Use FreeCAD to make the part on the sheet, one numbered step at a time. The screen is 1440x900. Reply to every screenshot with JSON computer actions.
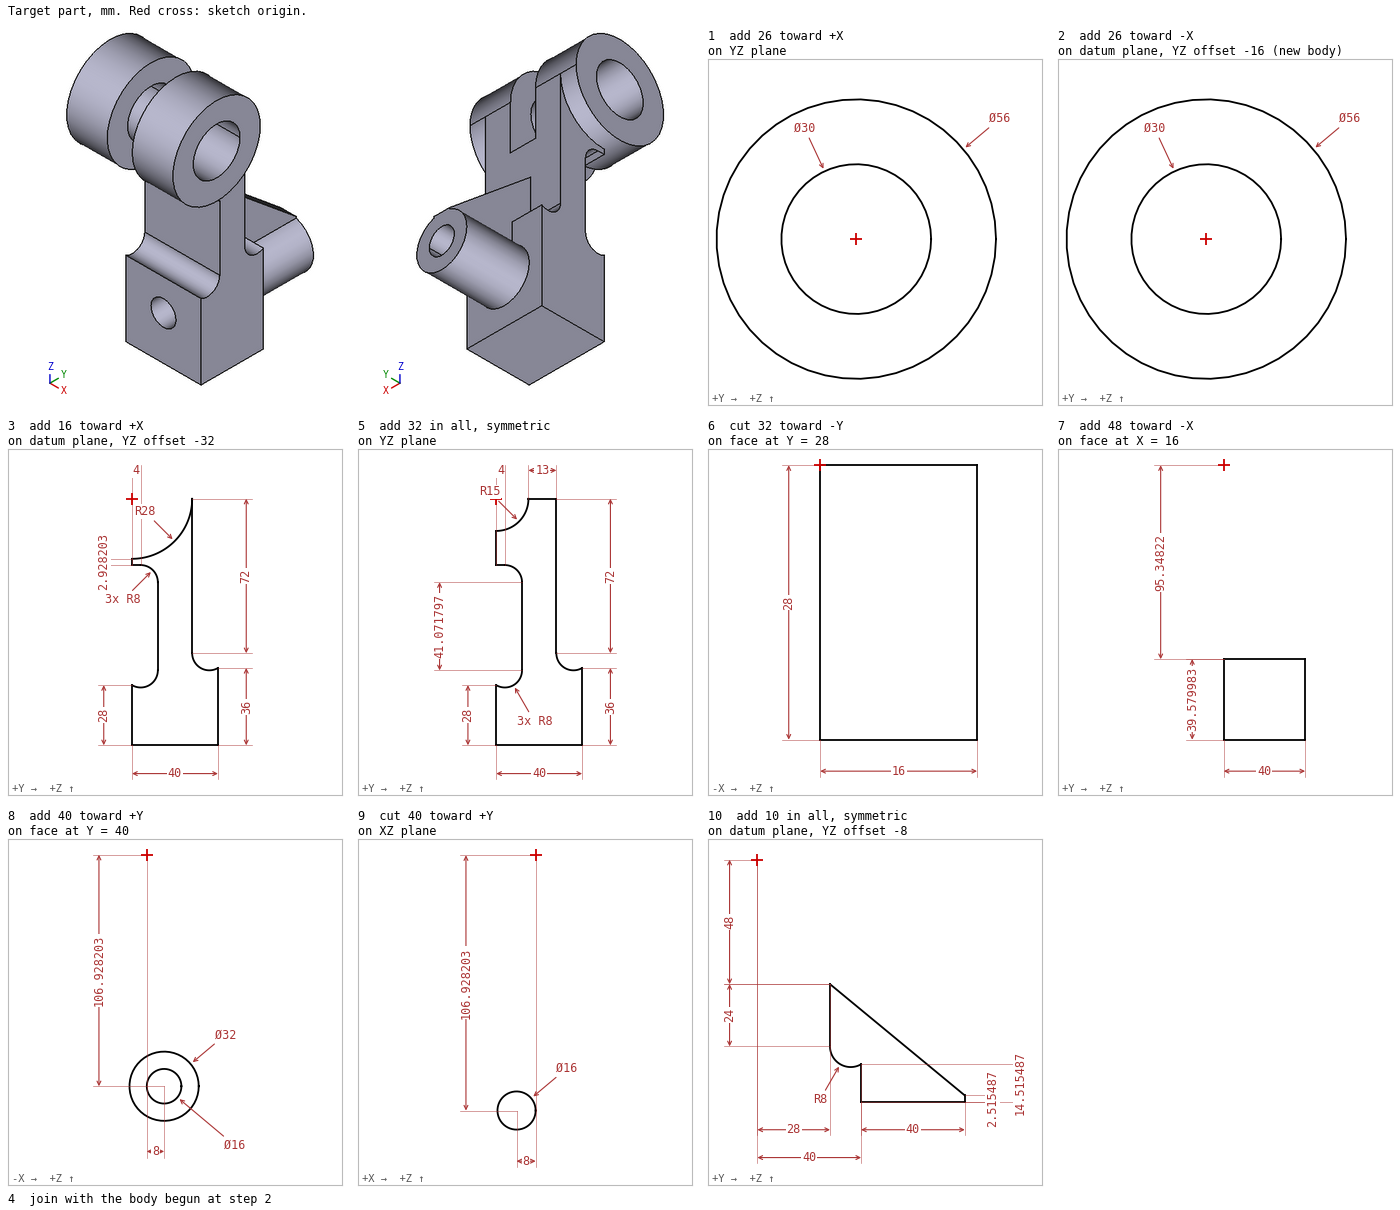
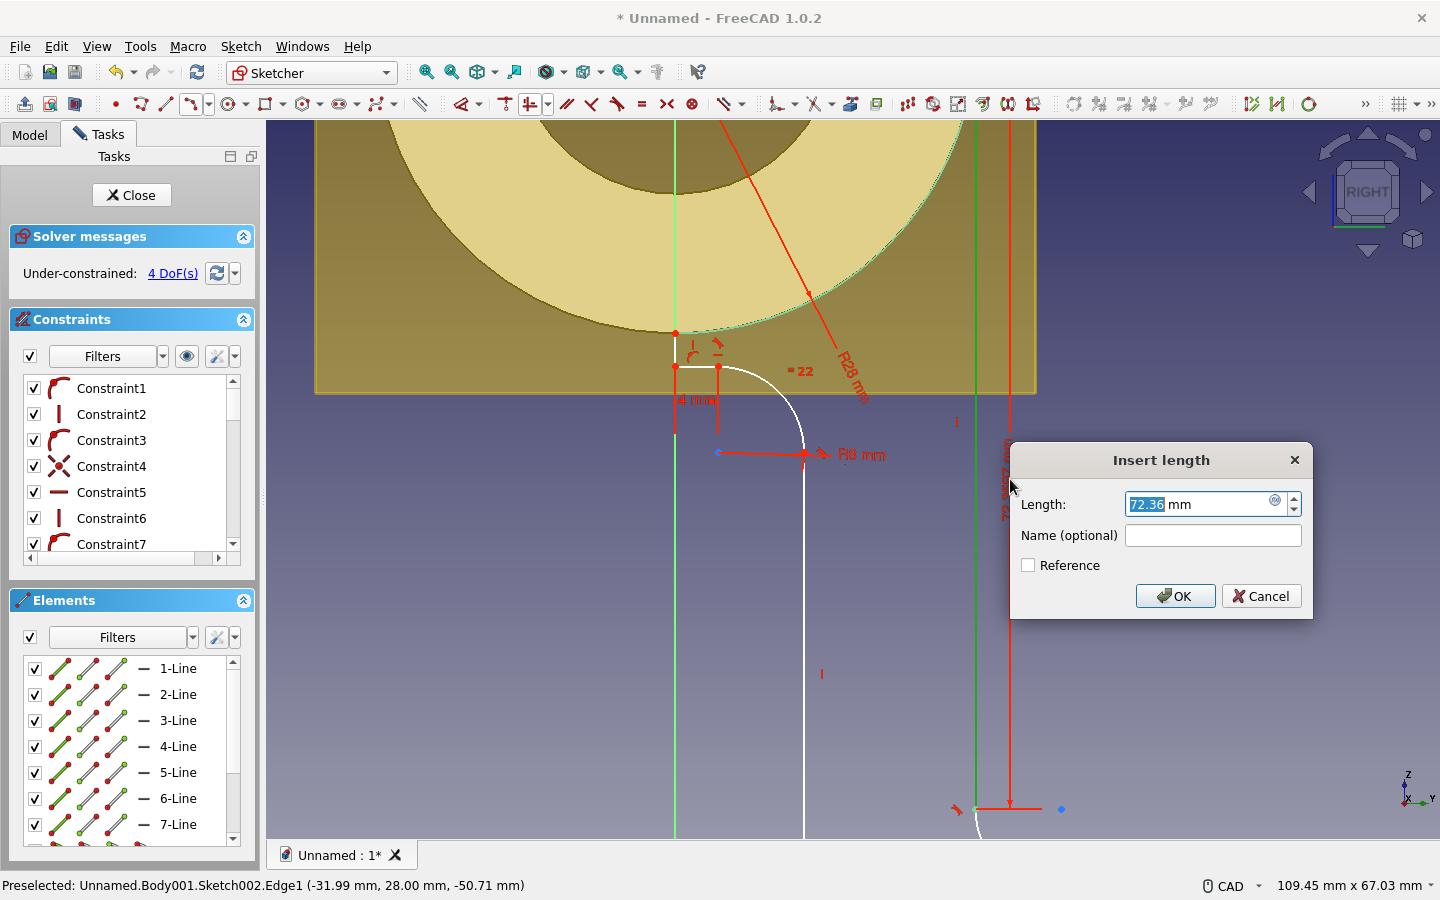
{"action": "type", "text": "72"}
{"action": "key", "text": "Return"}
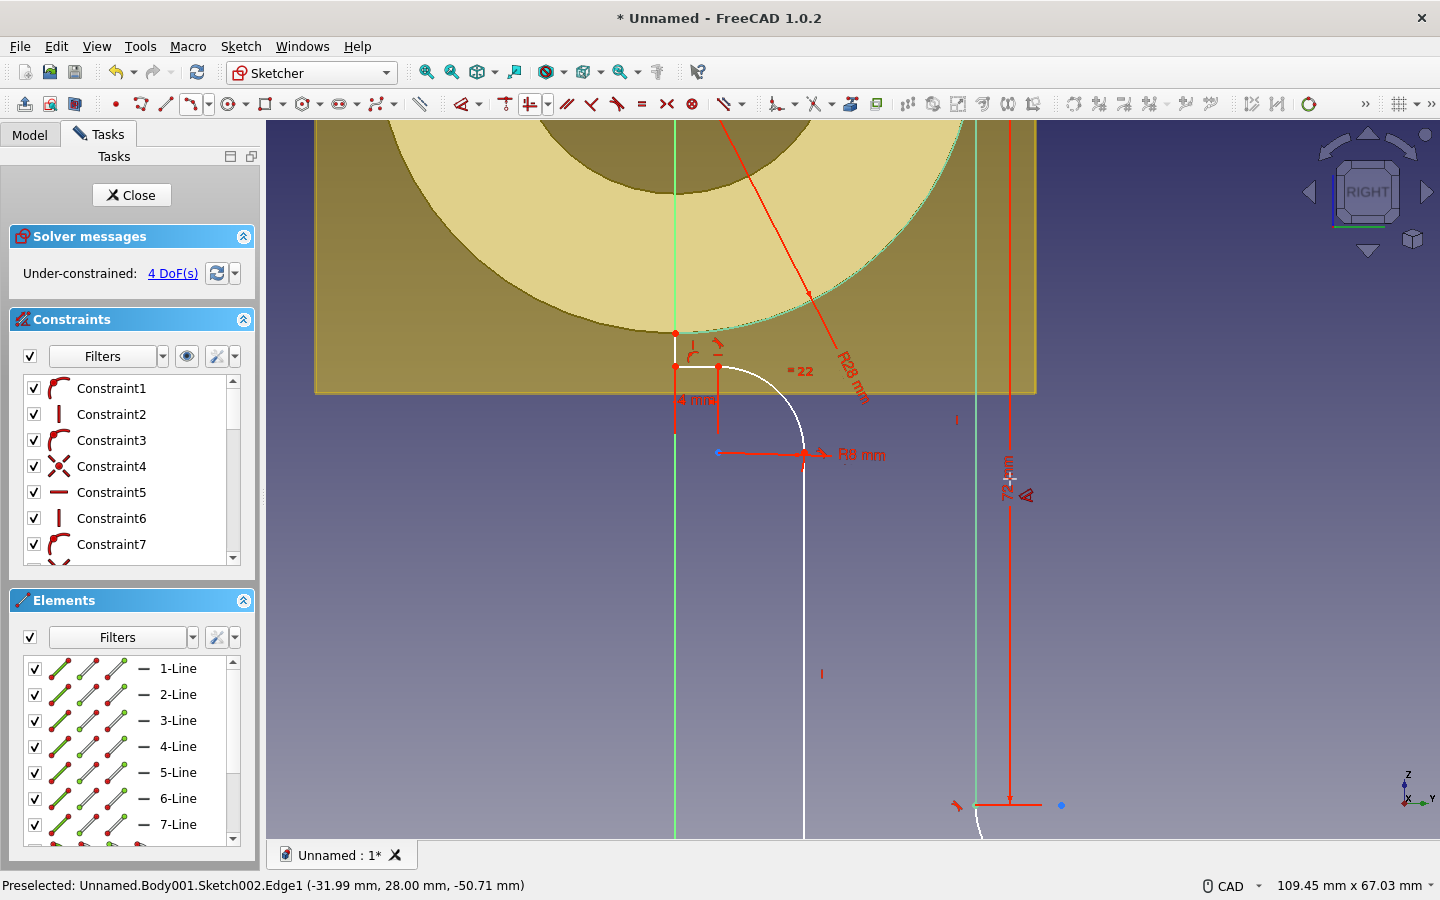
{"action": "scroll", "coordinate": [723, 381], "scroll_direction": "down", "scroll_amount": 5}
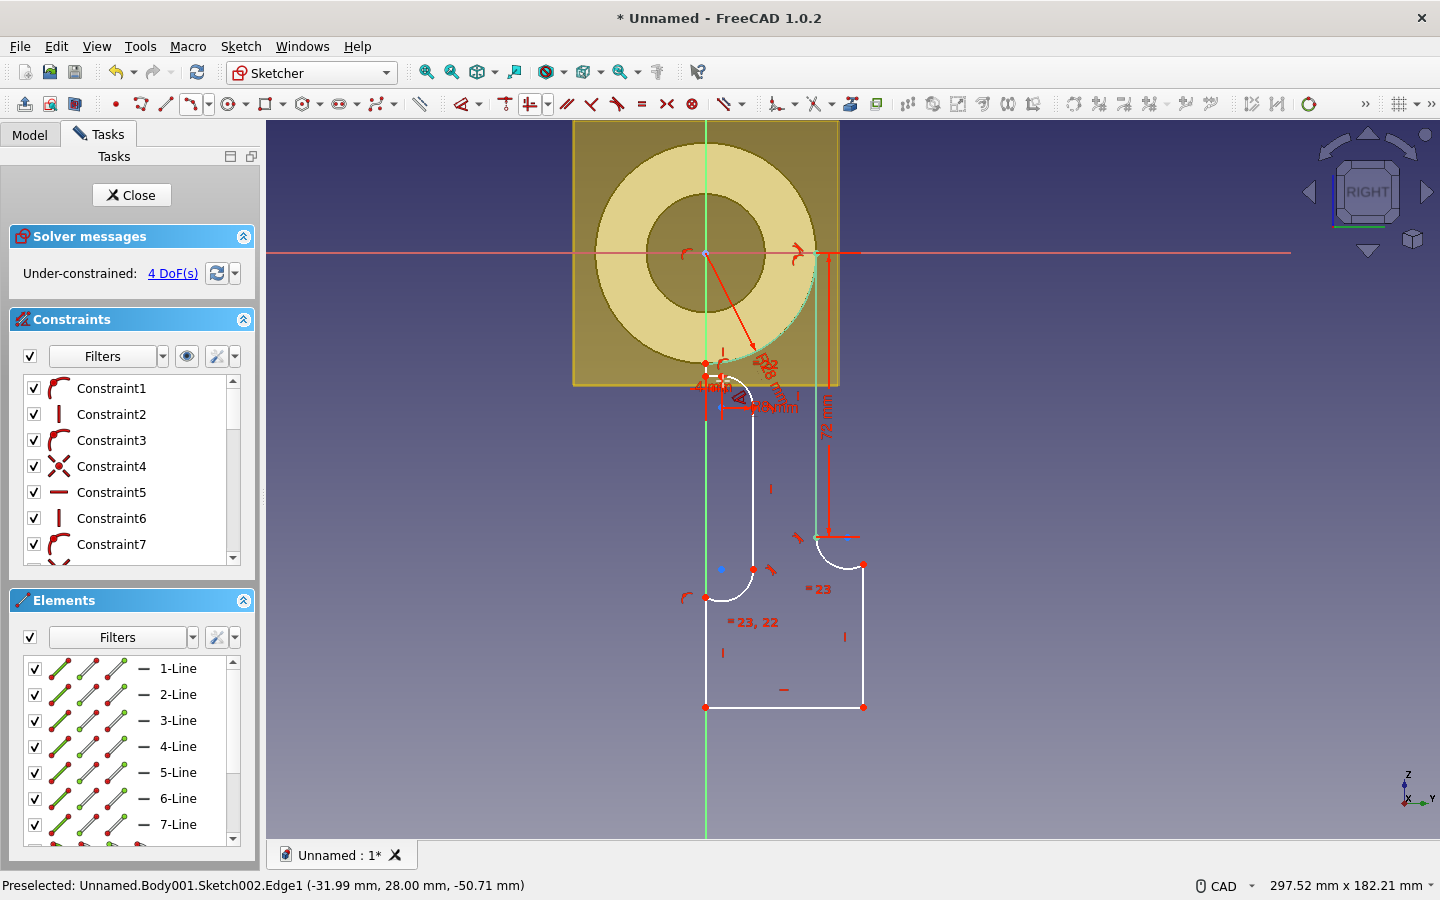
{"action": "left_click", "coordinate": [706, 630]}
{"action": "left_click", "coordinate": [672, 652]}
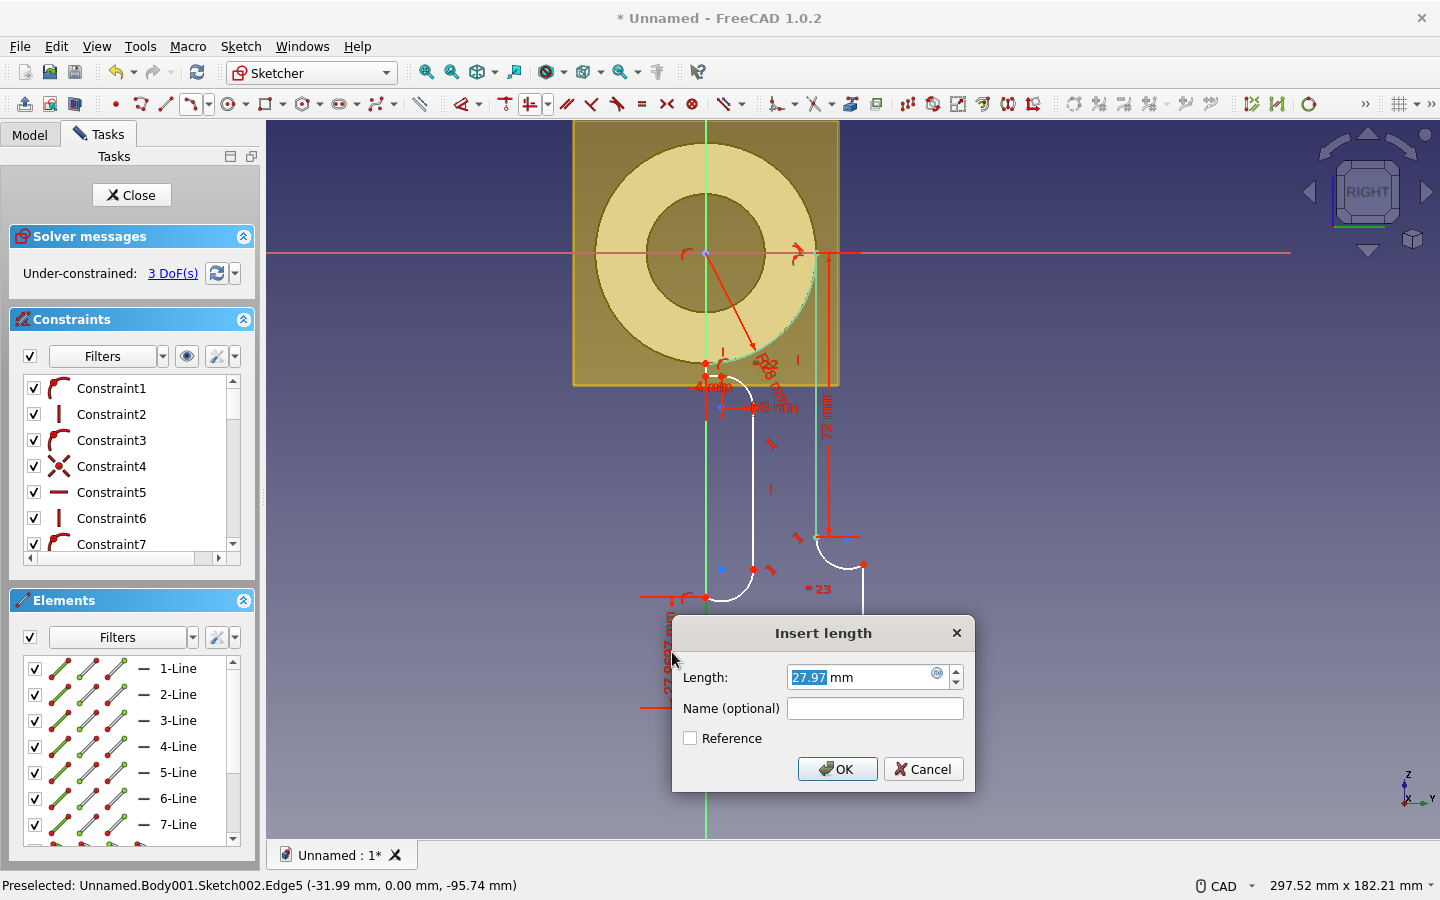
{"action": "type", "text": "28"}
{"action": "key", "text": "Return"}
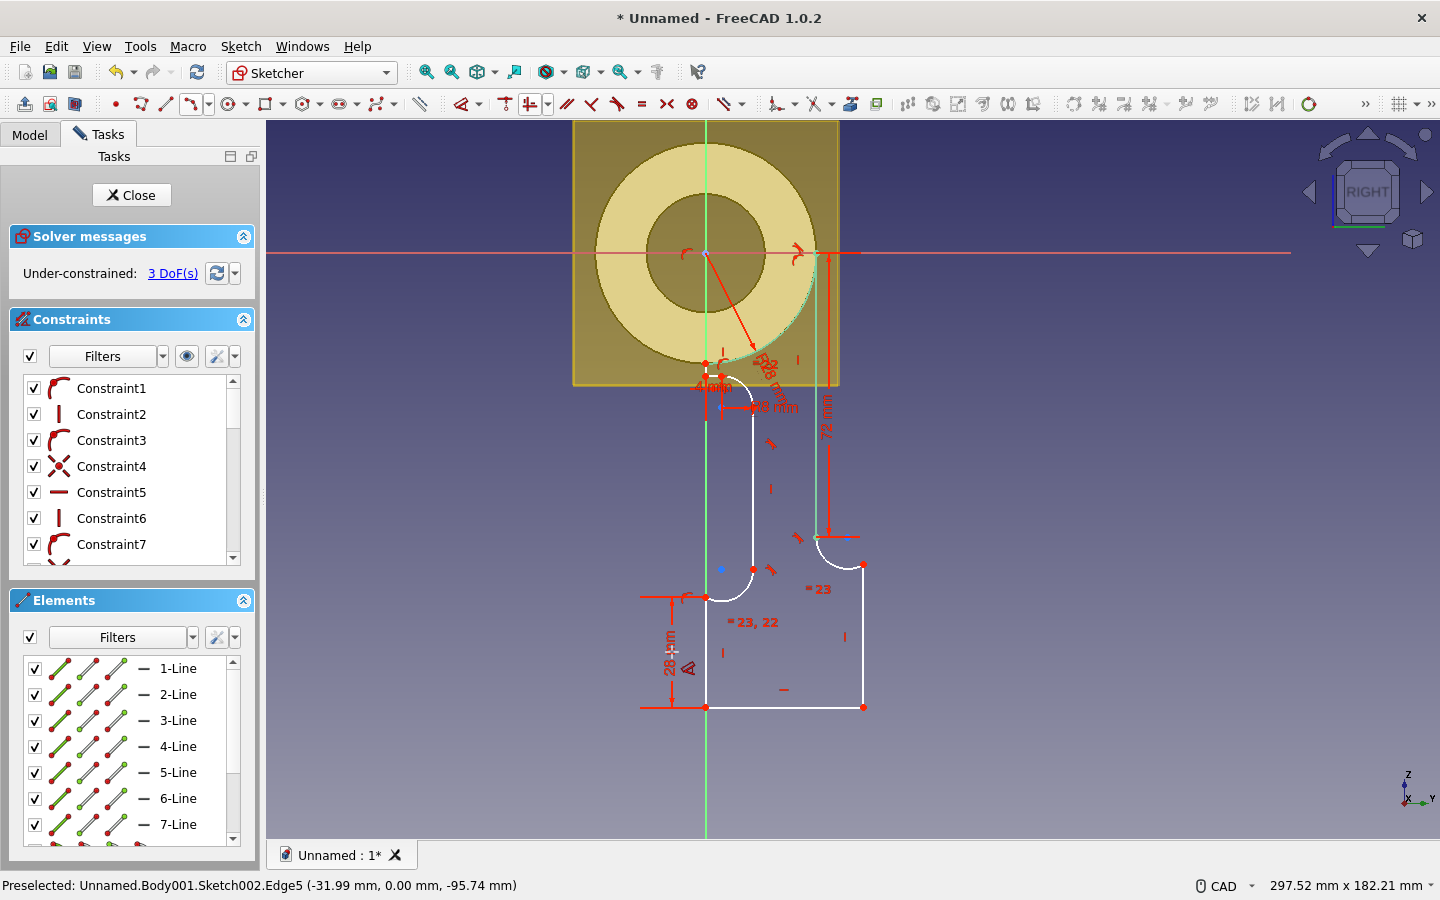
{"action": "left_click", "coordinate": [753, 708]}
{"action": "left_click", "coordinate": [784, 742]}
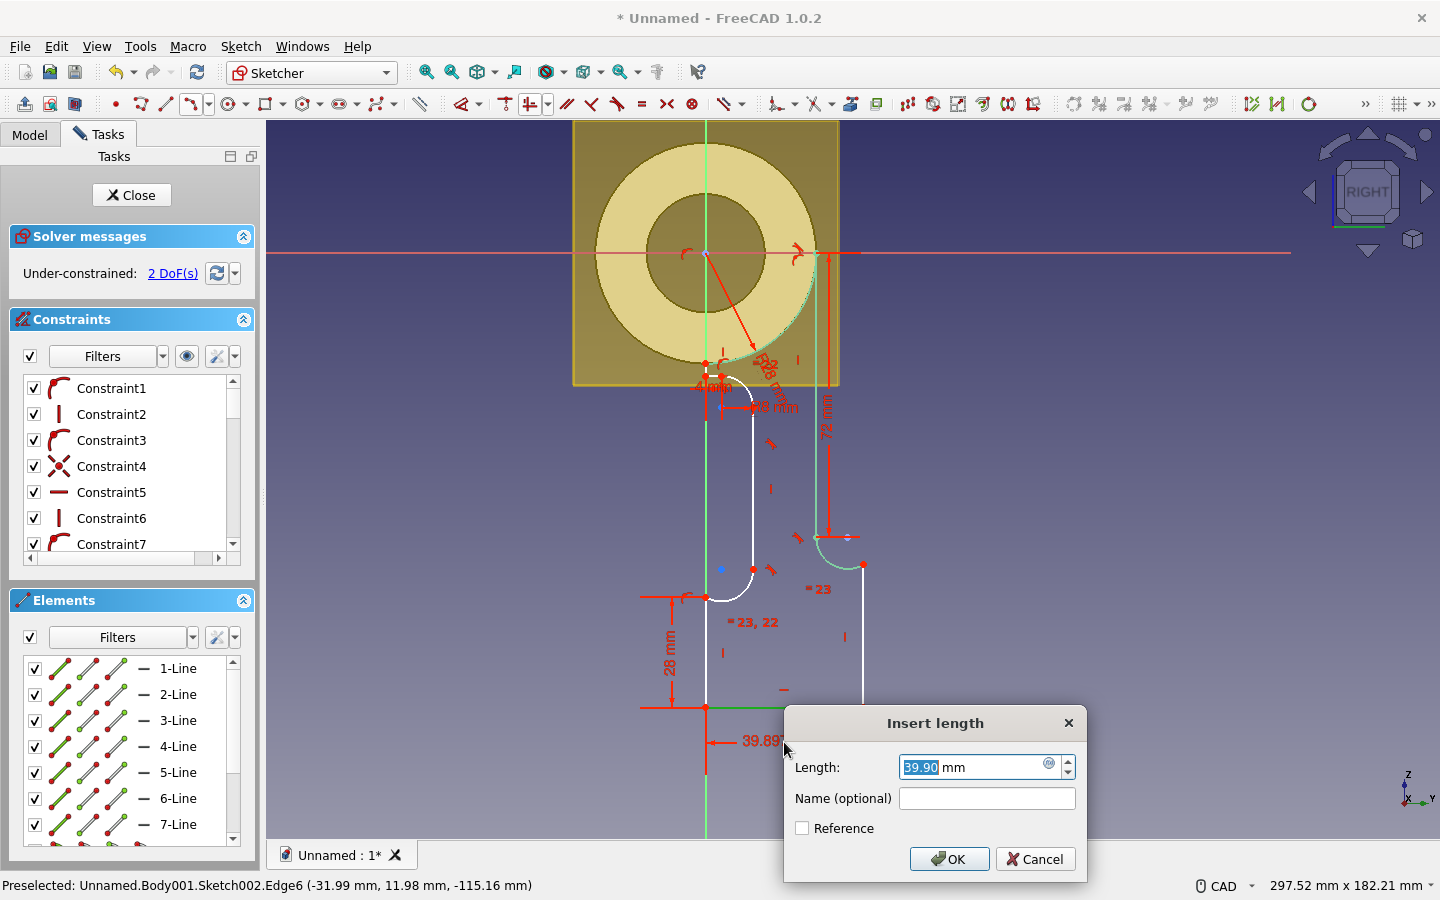
{"action": "type", "text": "40"}
{"action": "key", "text": "Return"}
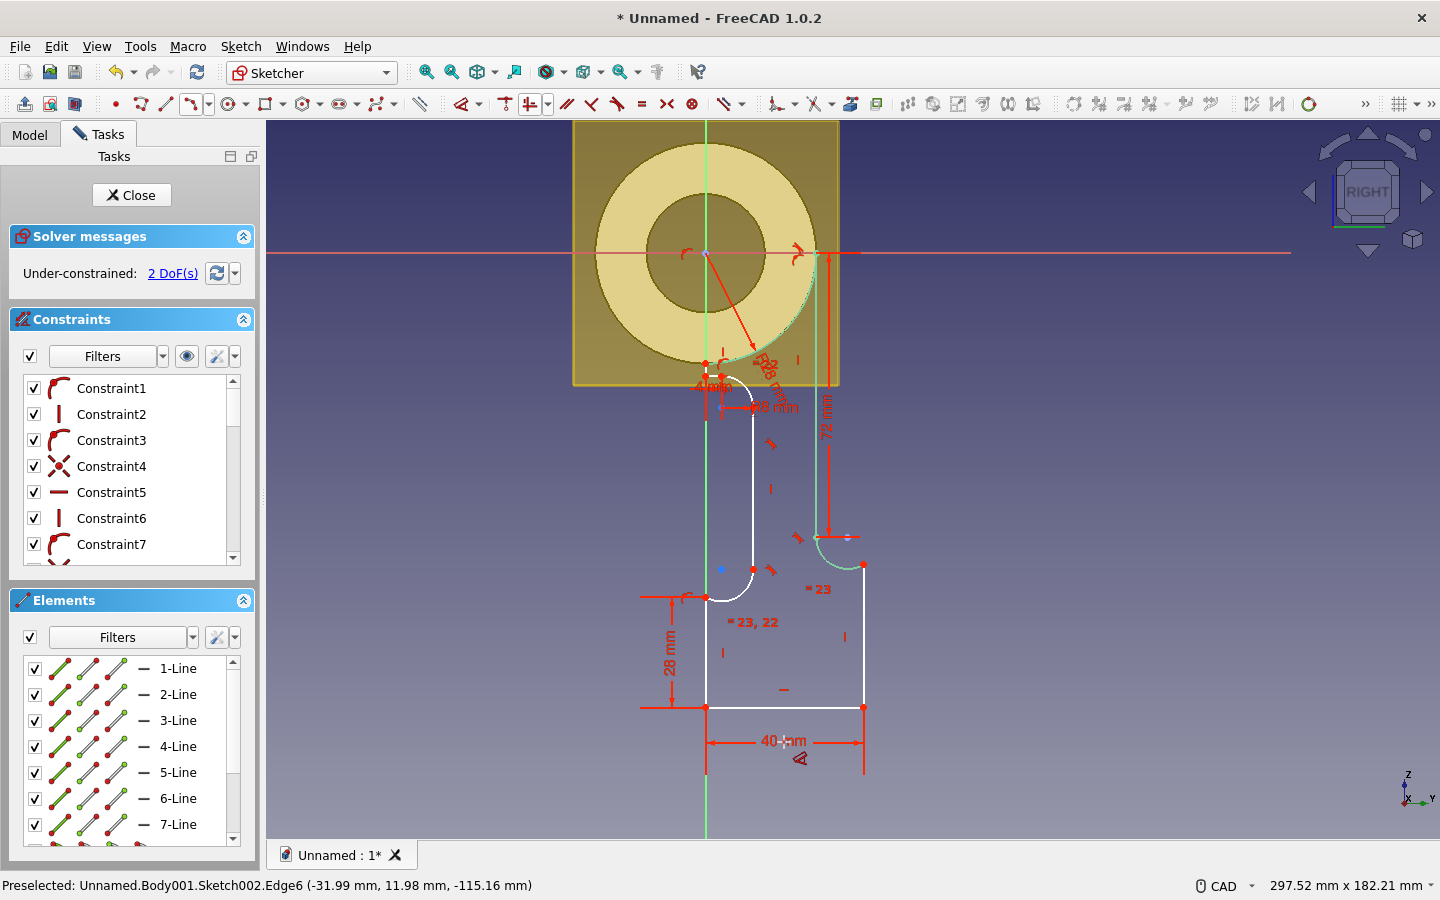
{"action": "left_click", "coordinate": [864, 665]}
{"action": "left_click", "coordinate": [898, 636]}